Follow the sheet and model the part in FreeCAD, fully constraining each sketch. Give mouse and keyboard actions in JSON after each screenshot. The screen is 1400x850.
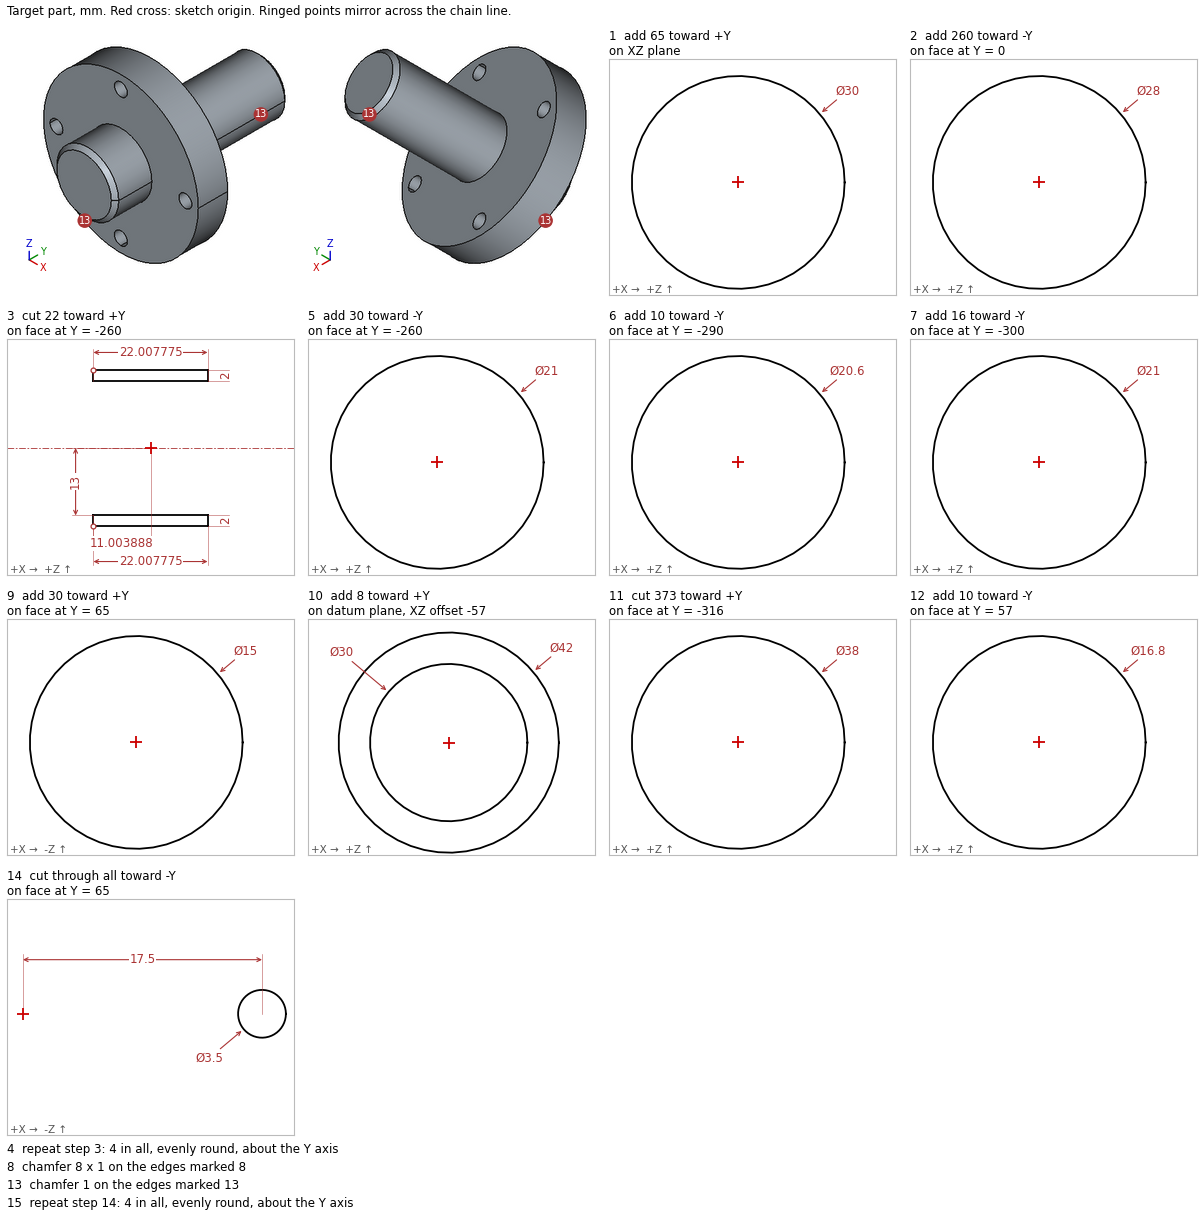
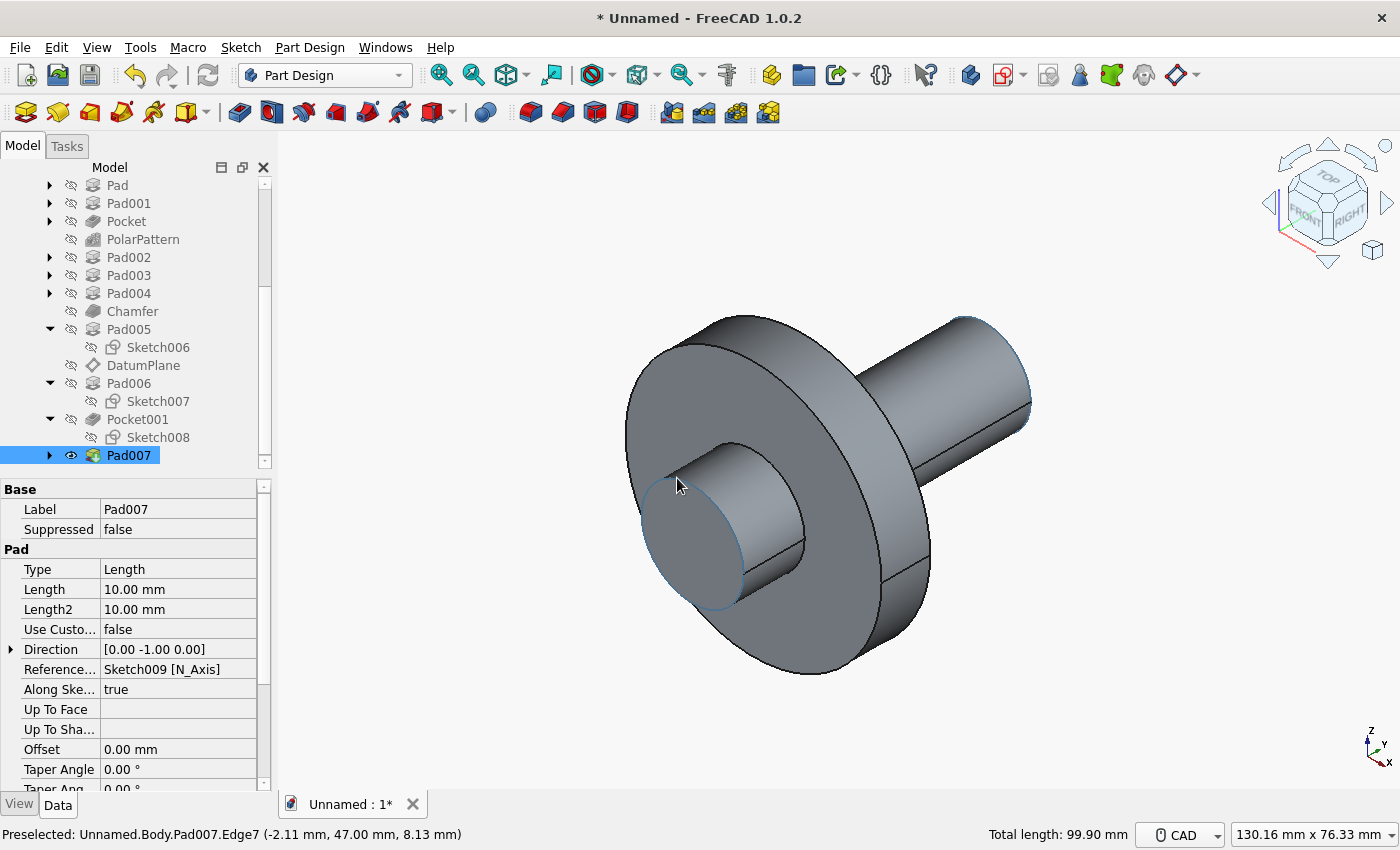
{"action": "left_click", "coordinate": [564, 112]}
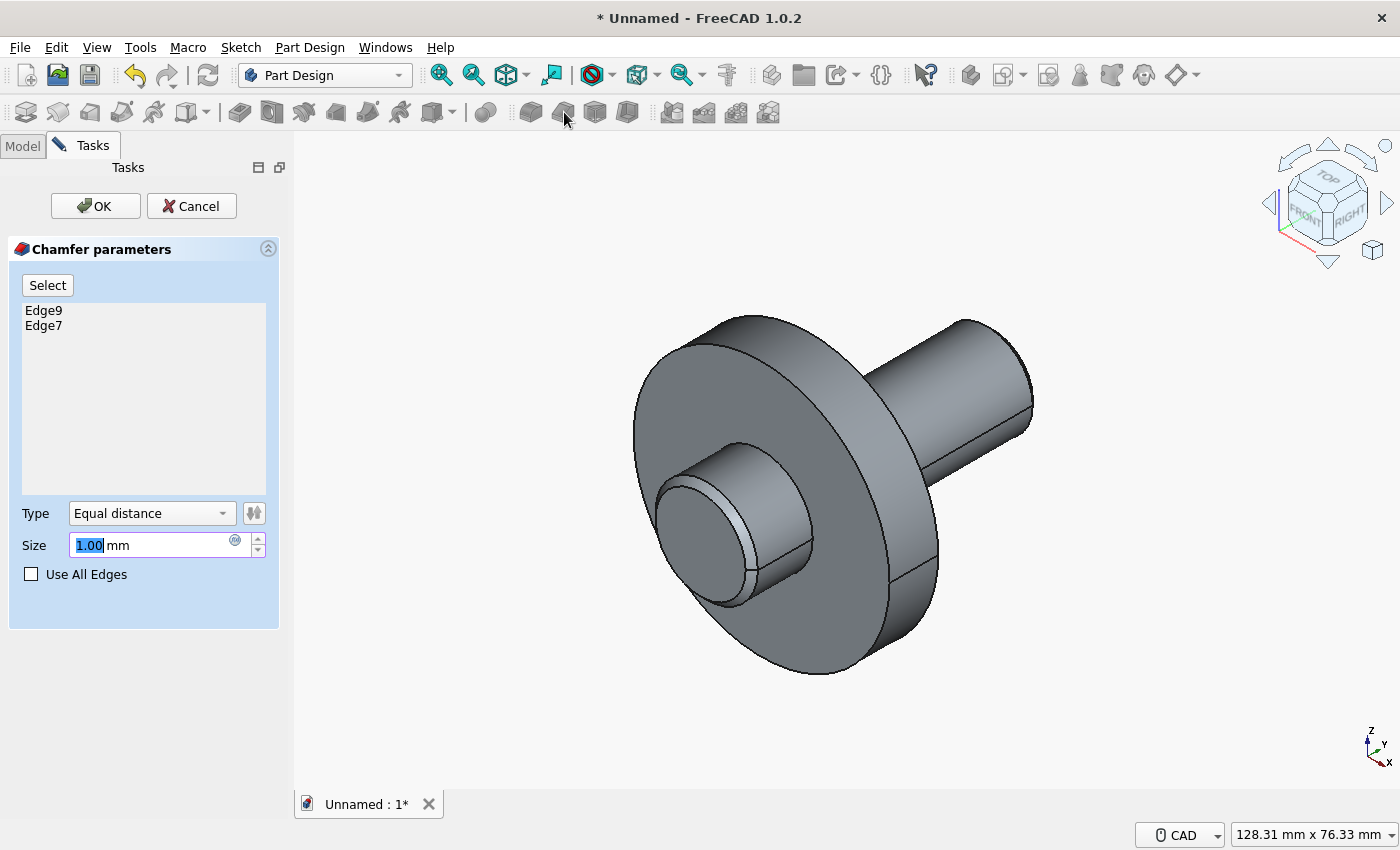
{"action": "type", "text": "1"}
{"action": "key", "text": "Tab"}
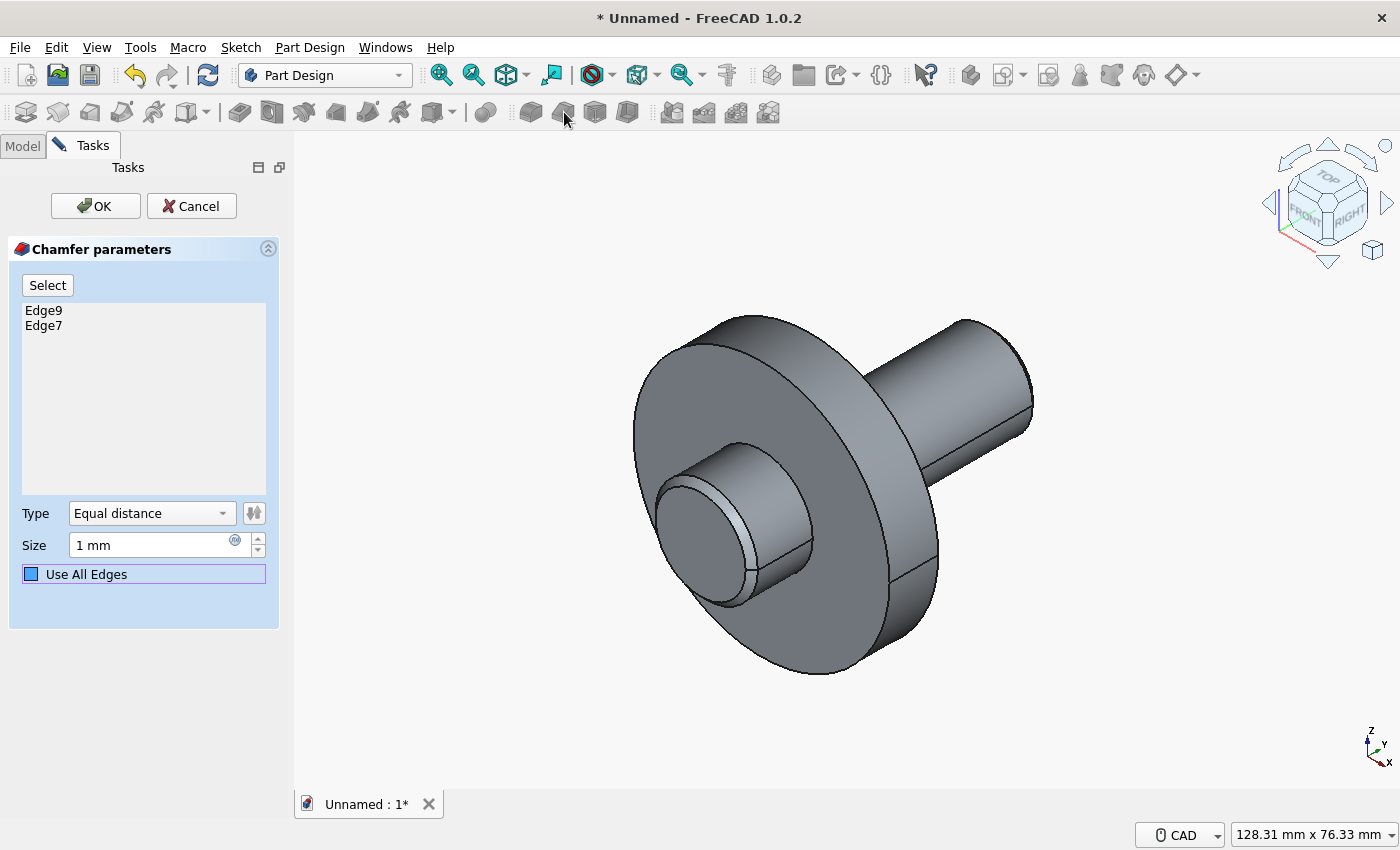
{"action": "left_click", "coordinate": [96, 206]}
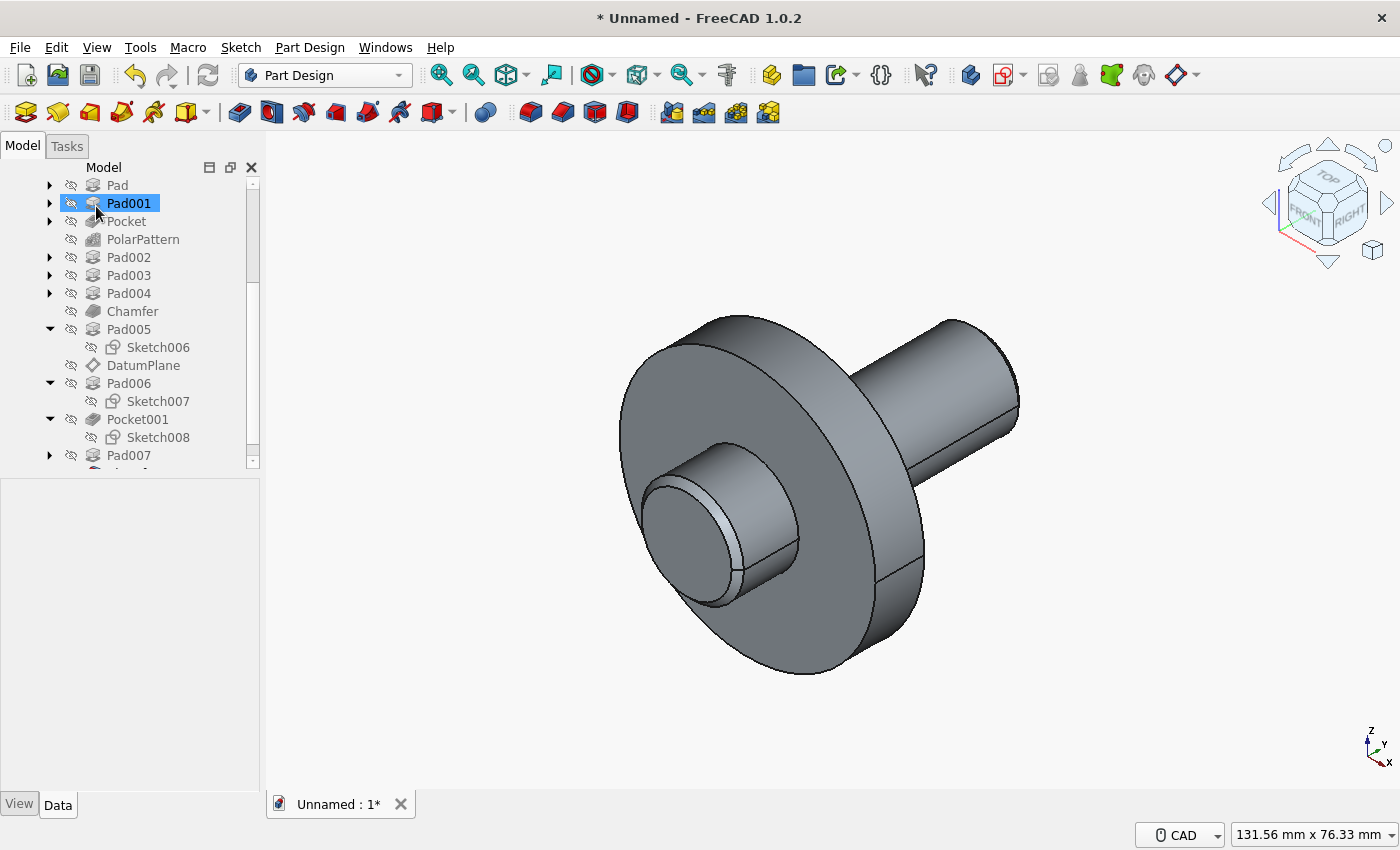
{"action": "key", "text": "4"}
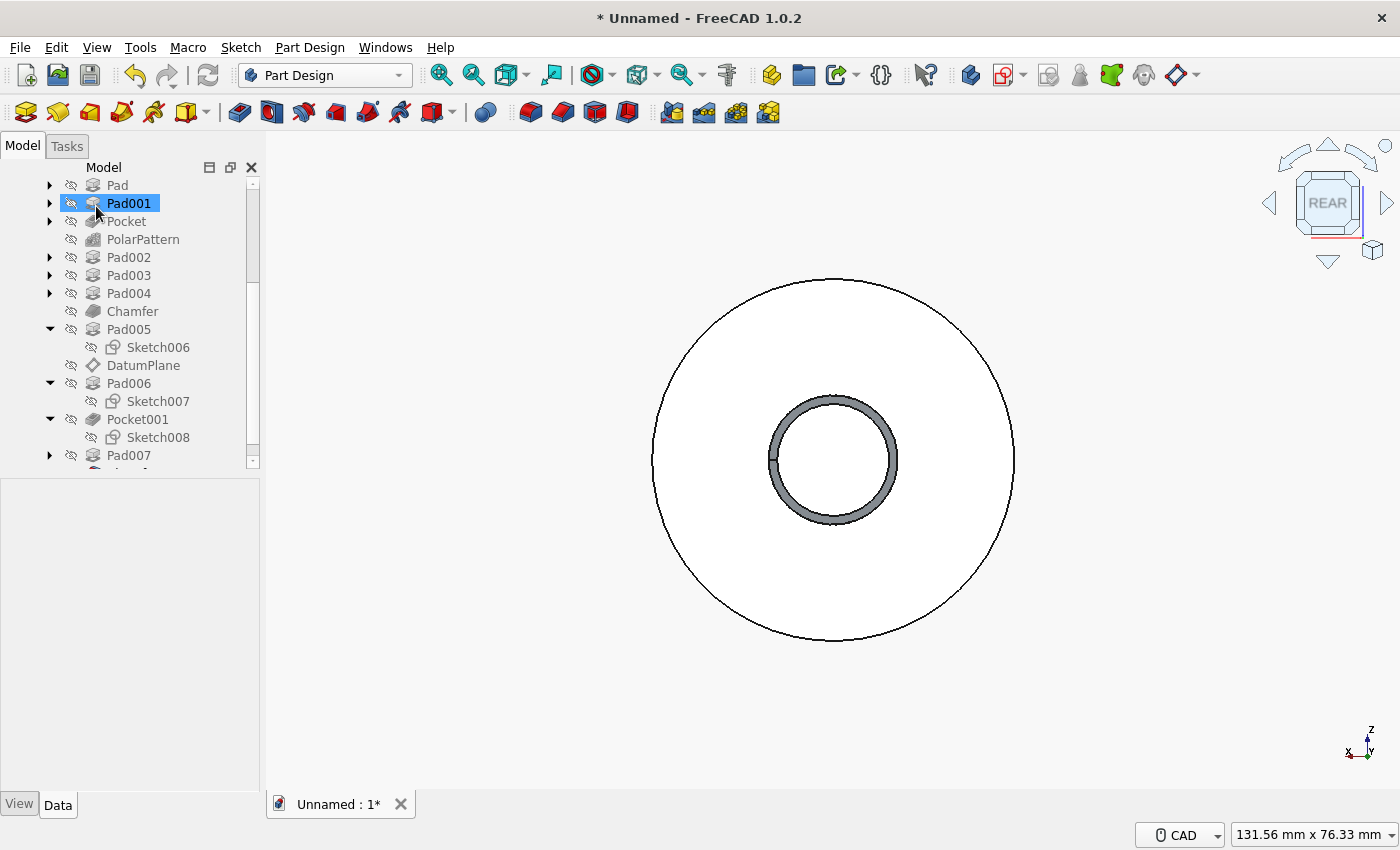
{"action": "left_click", "coordinate": [885, 562]}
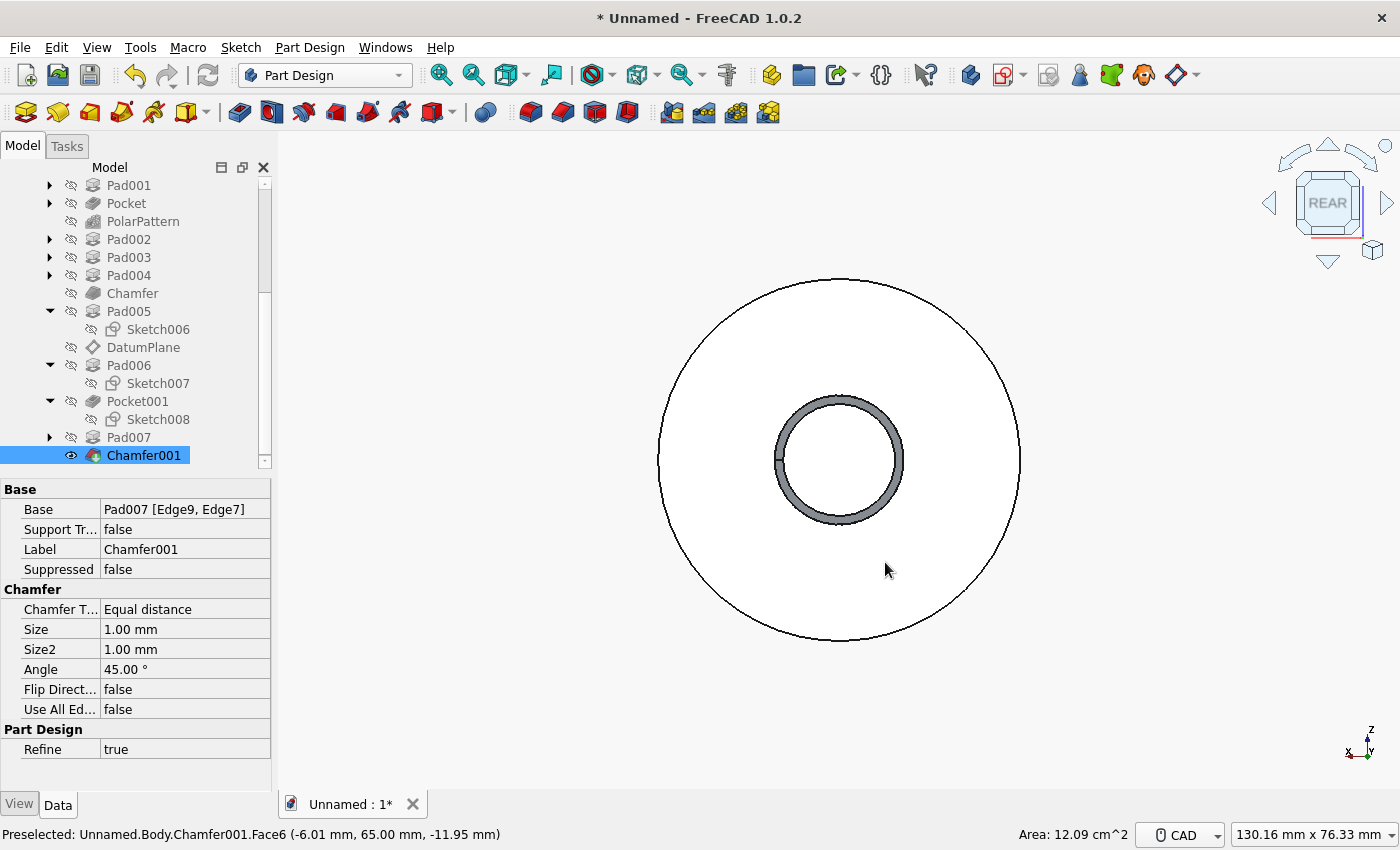
{"action": "left_click", "coordinate": [1004, 76]}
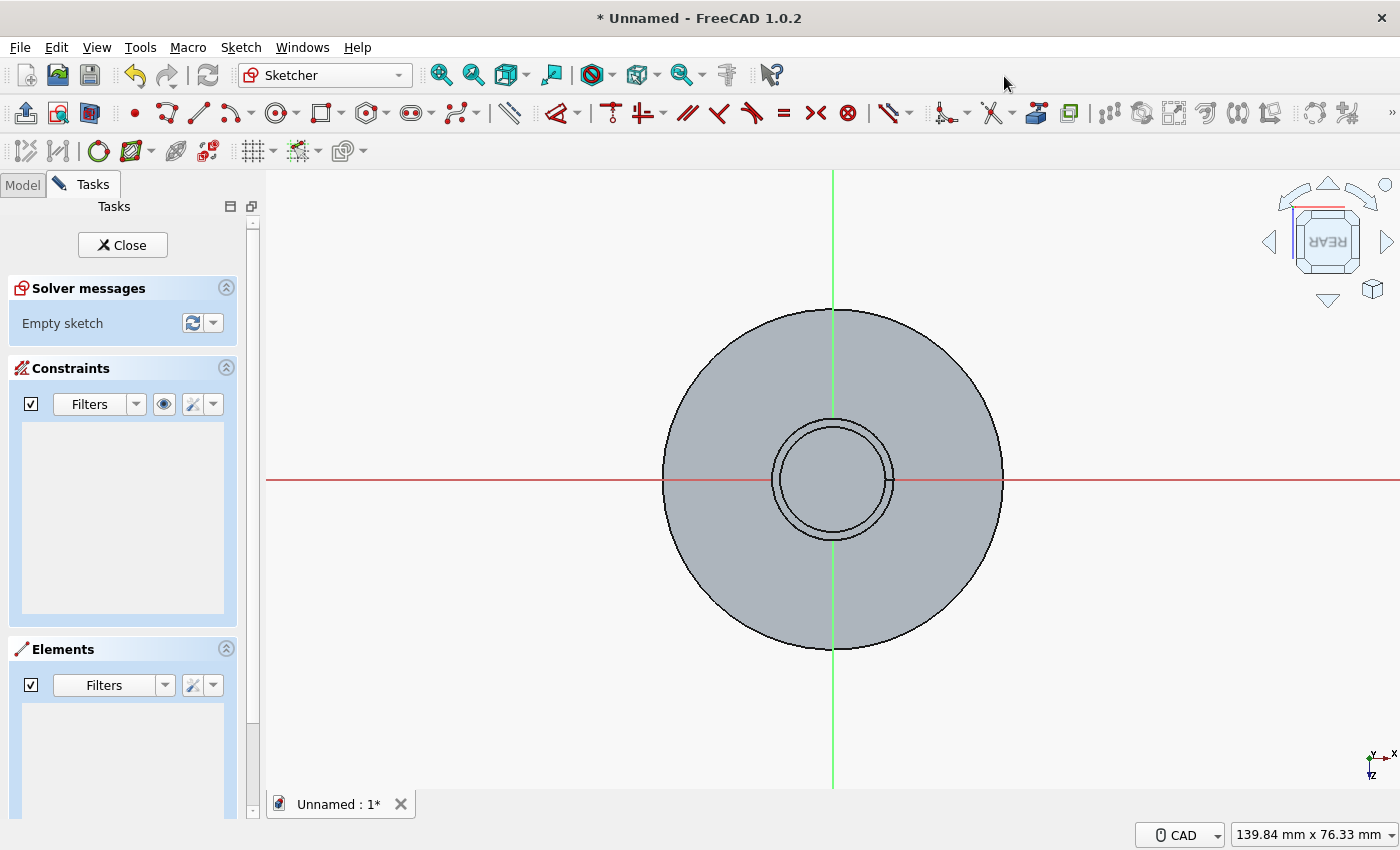
{"action": "left_click", "coordinate": [90, 114]}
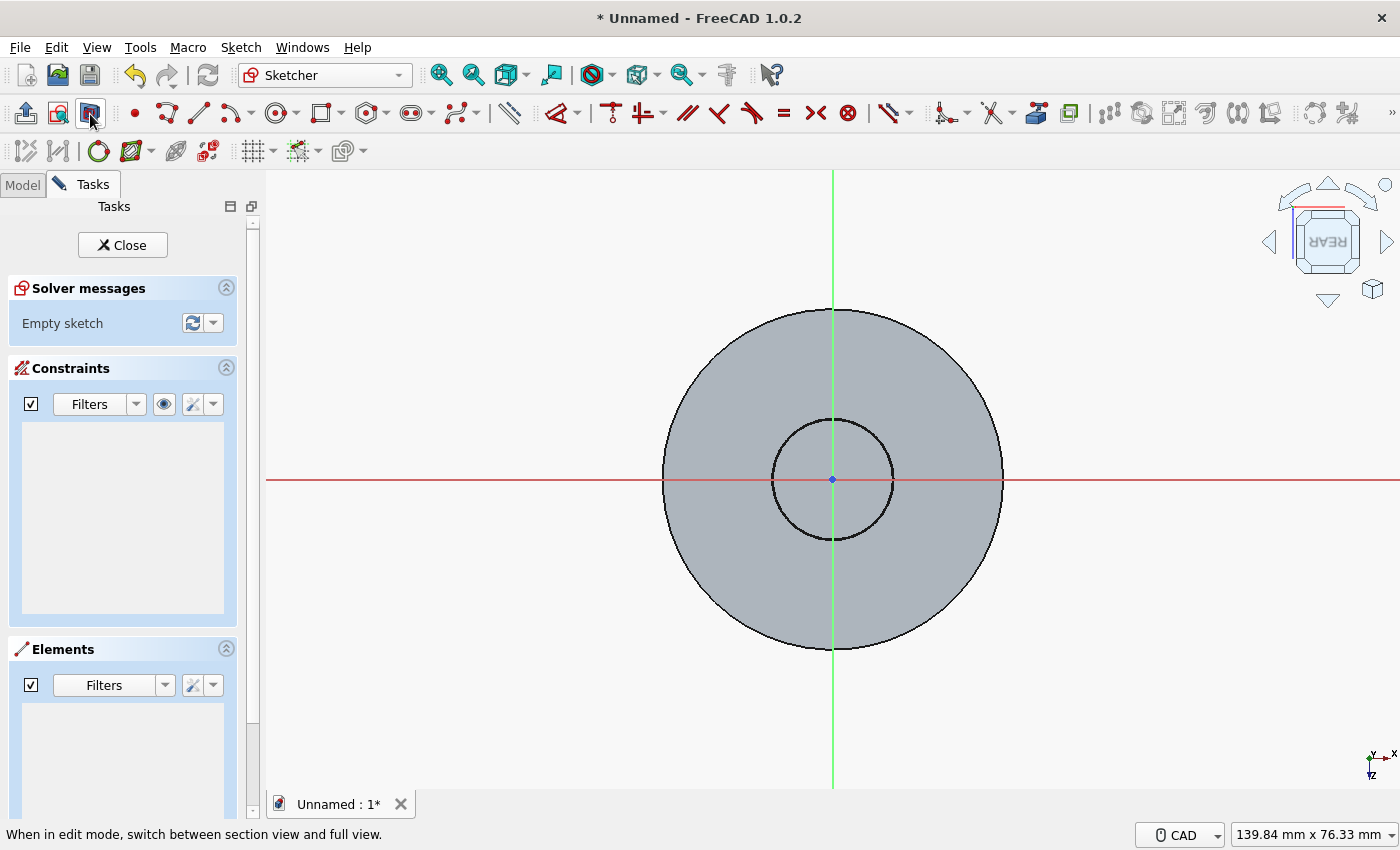
{"action": "scroll", "coordinate": [992, 479], "scroll_direction": "up", "scroll_amount": 13}